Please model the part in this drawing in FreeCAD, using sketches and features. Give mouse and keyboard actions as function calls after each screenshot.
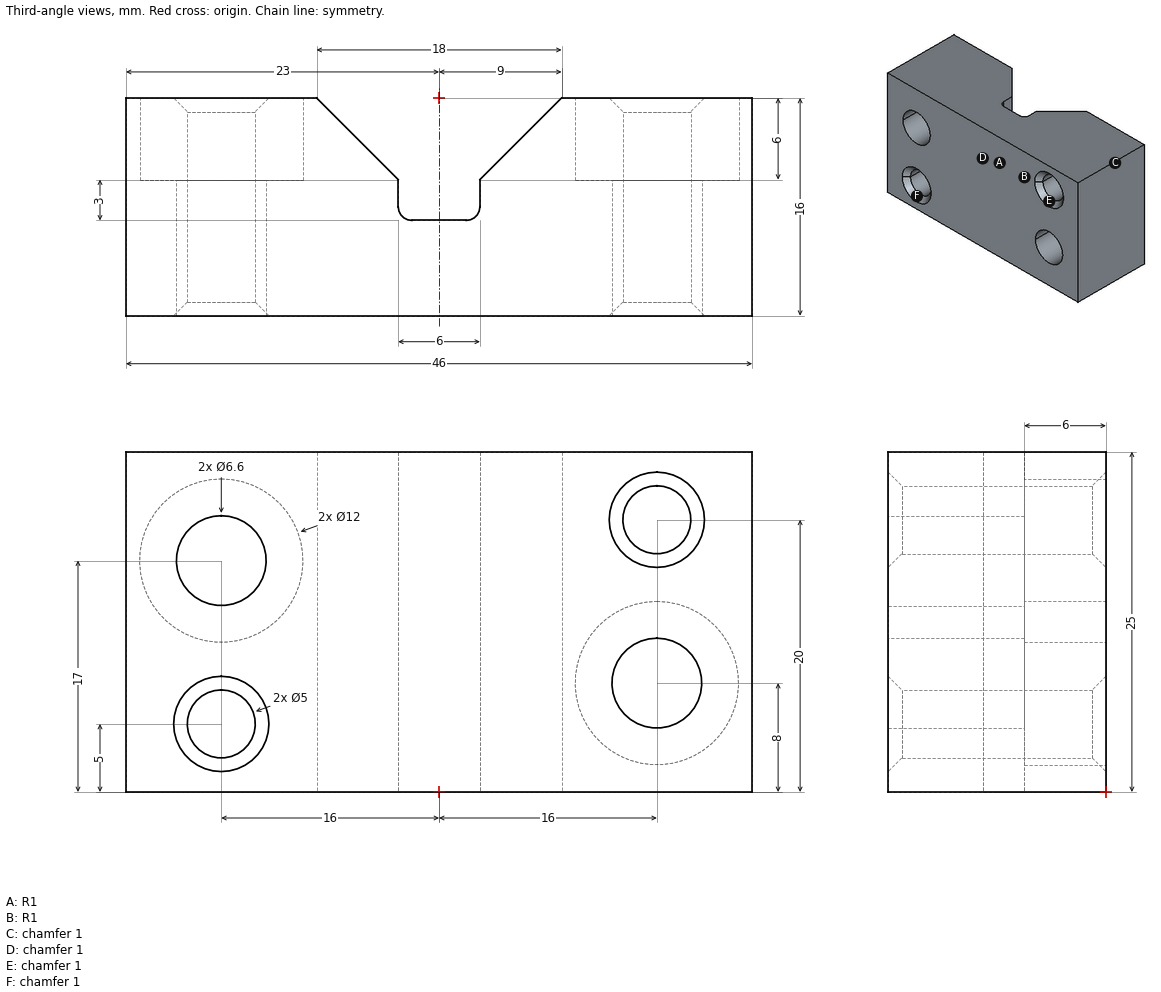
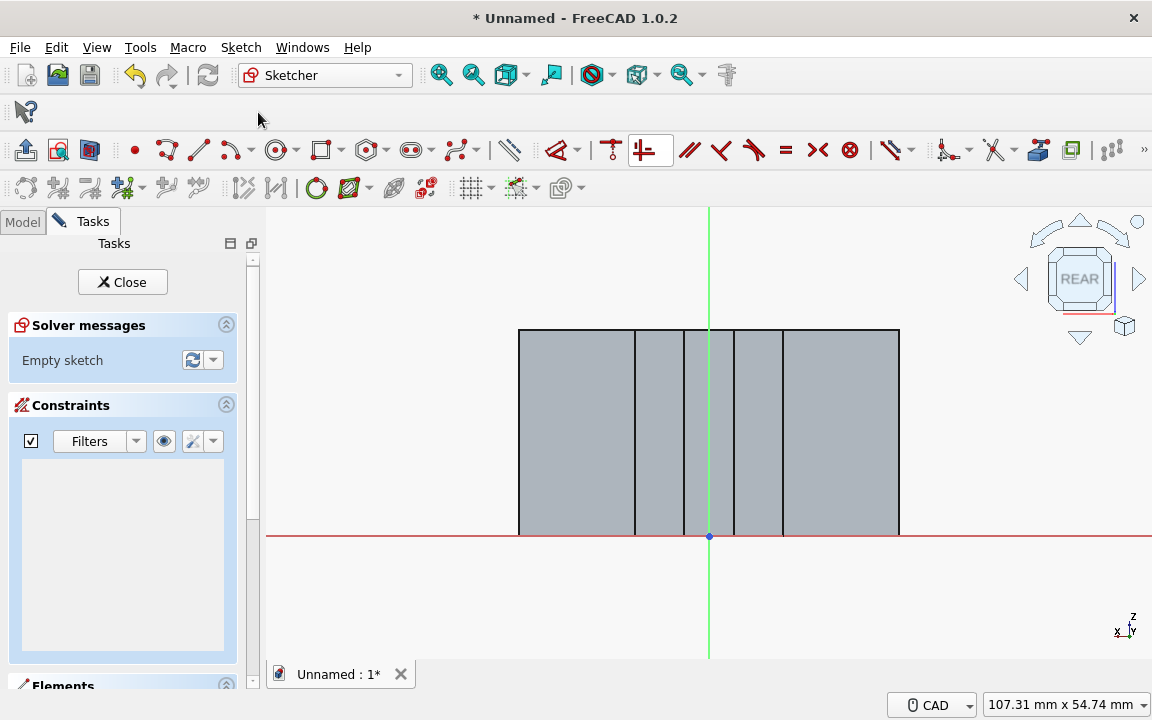
scroll(848, 464, up, 2)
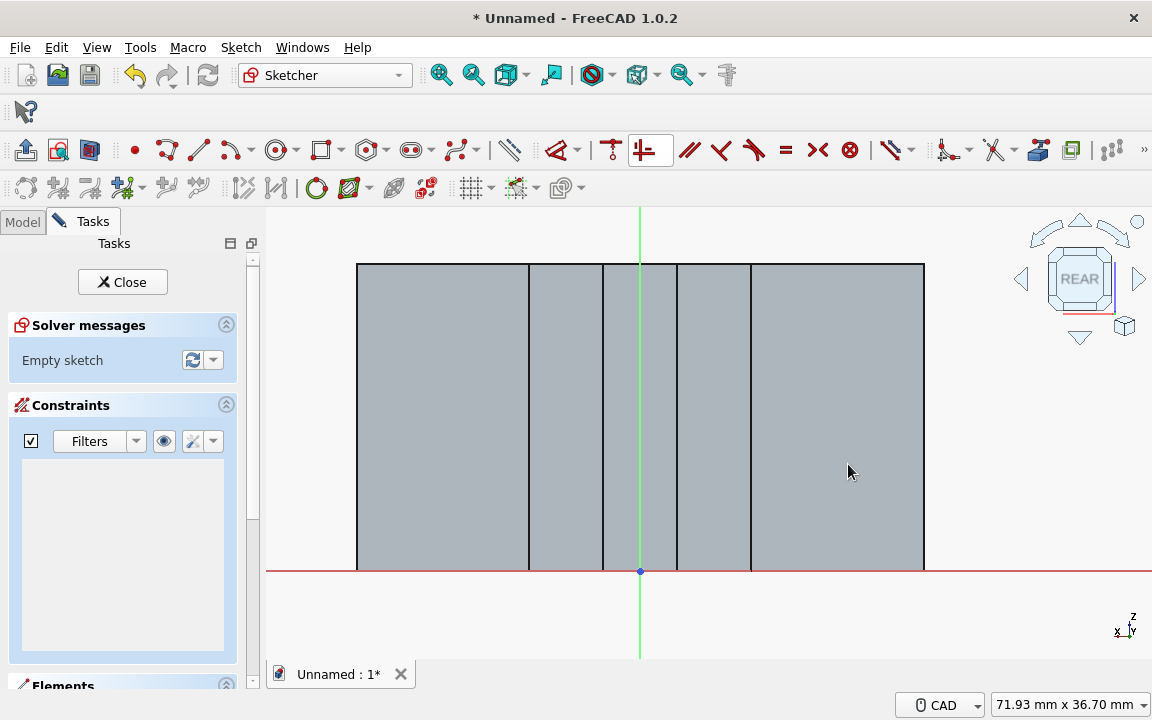
click(276, 150)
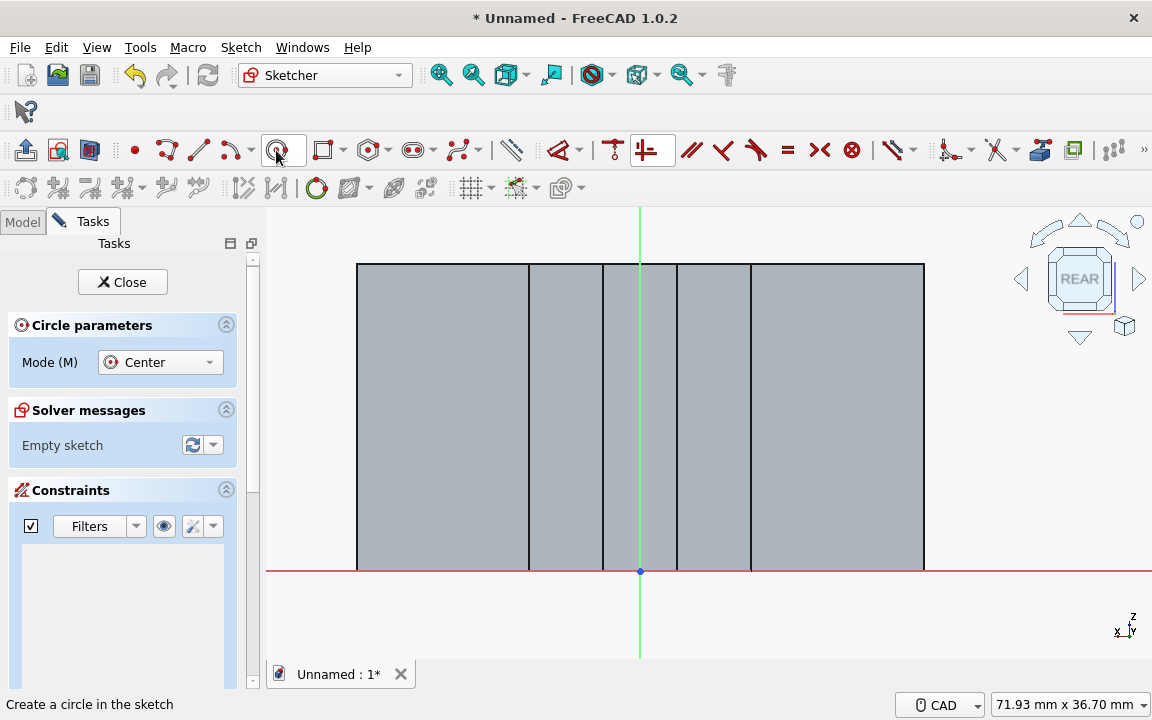
click(837, 362)
move(866, 333)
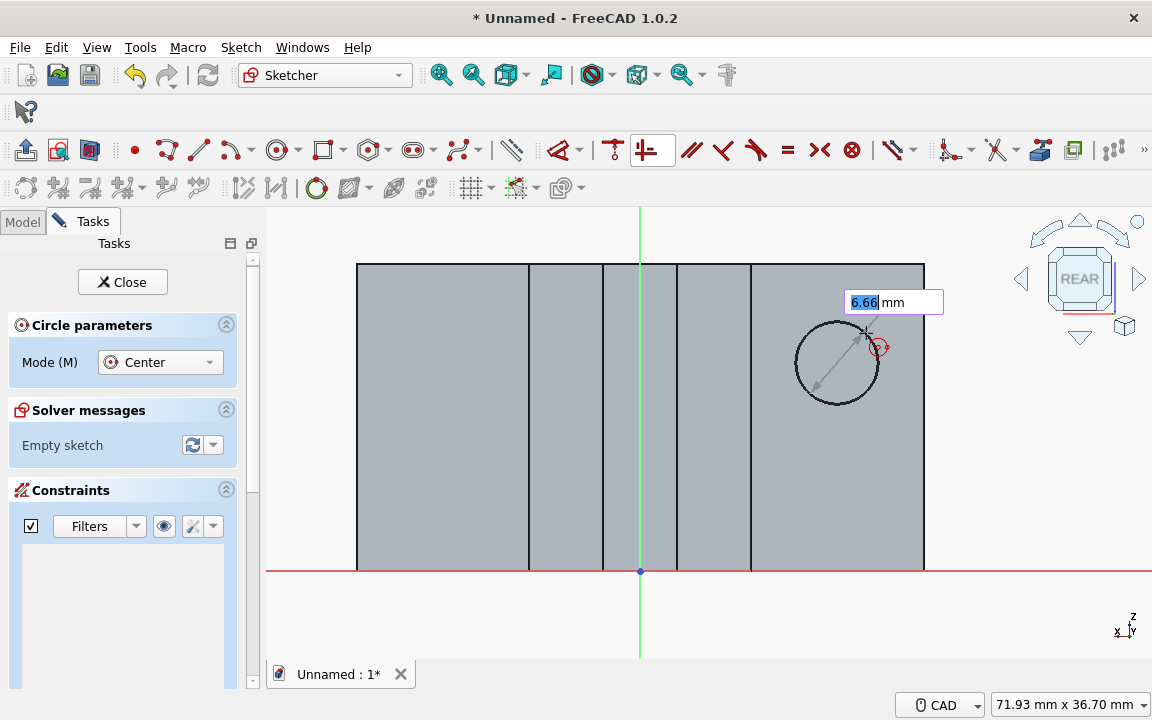
text(6.6)
key(Return)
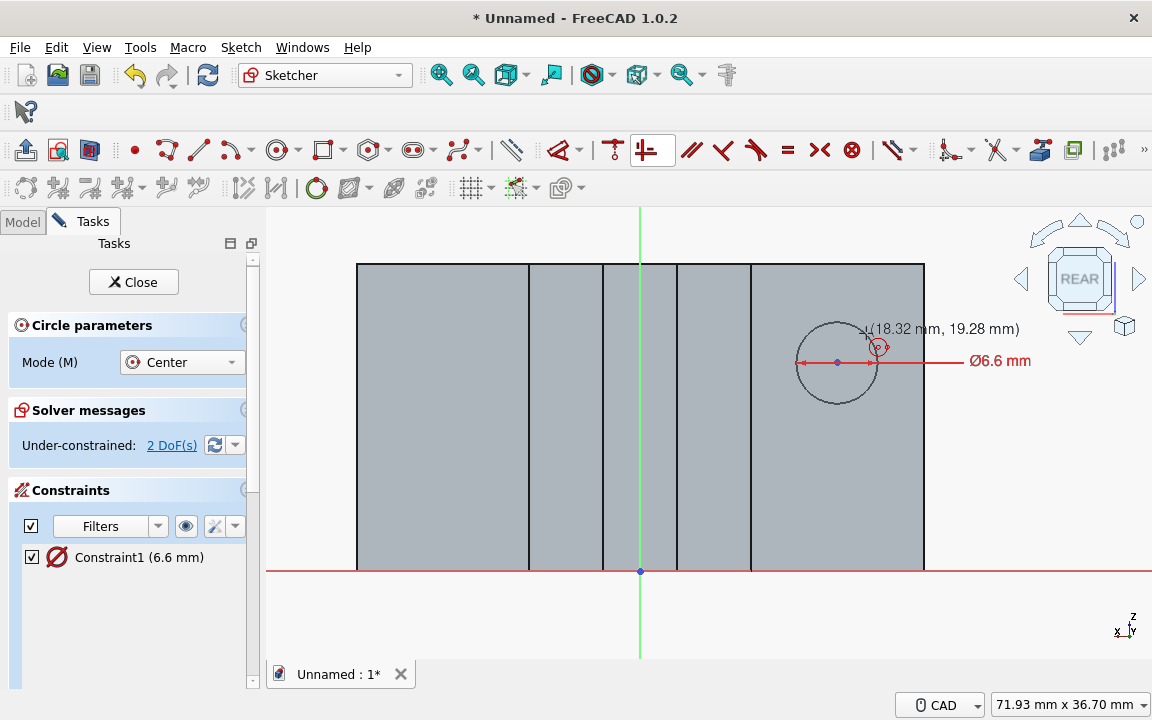
click(837, 510)
move(859, 488)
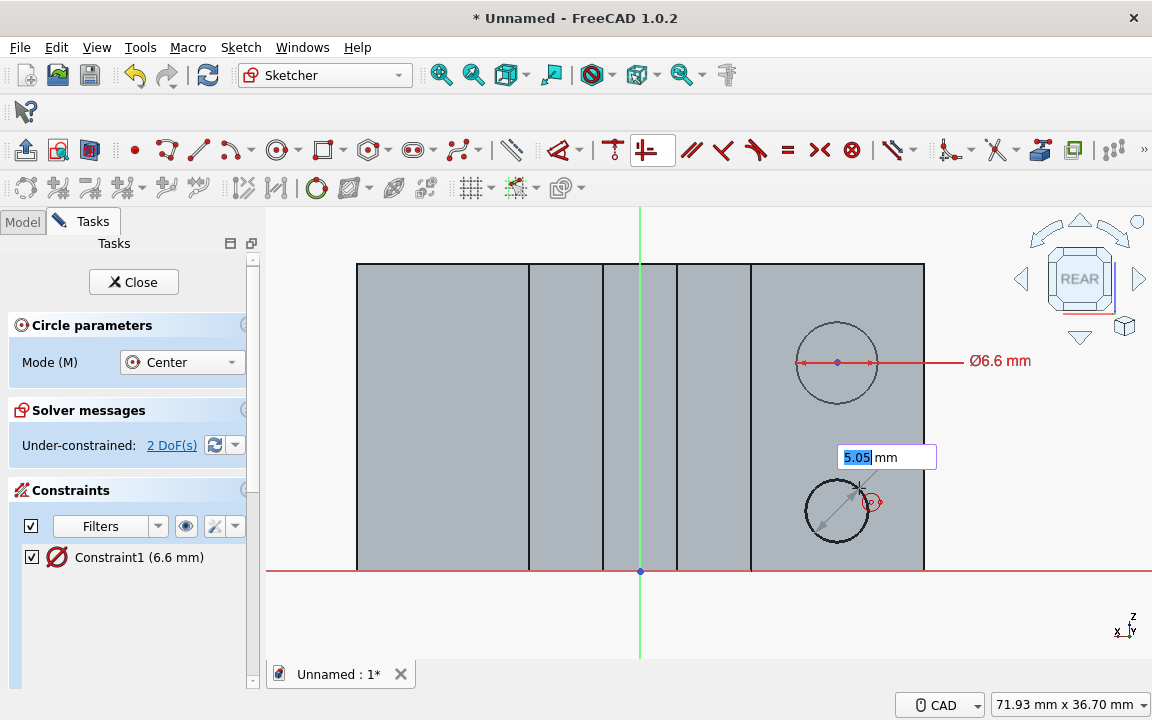
text(5)
key(Return)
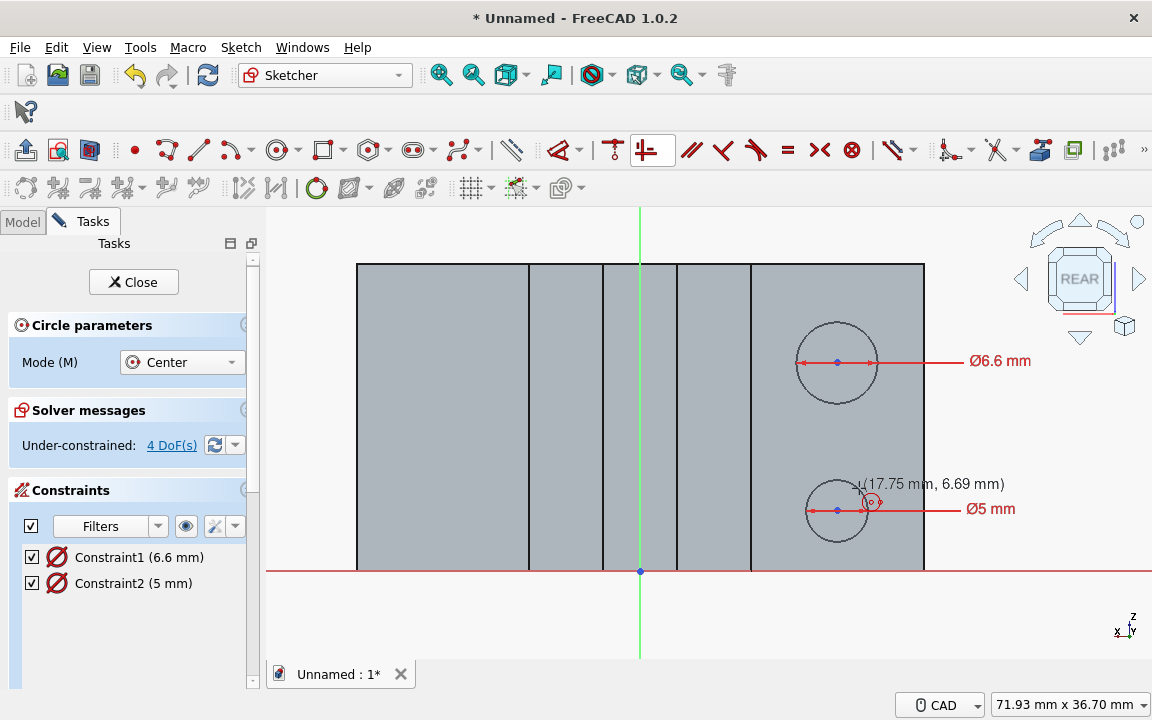
click(443, 325)
move(465, 303)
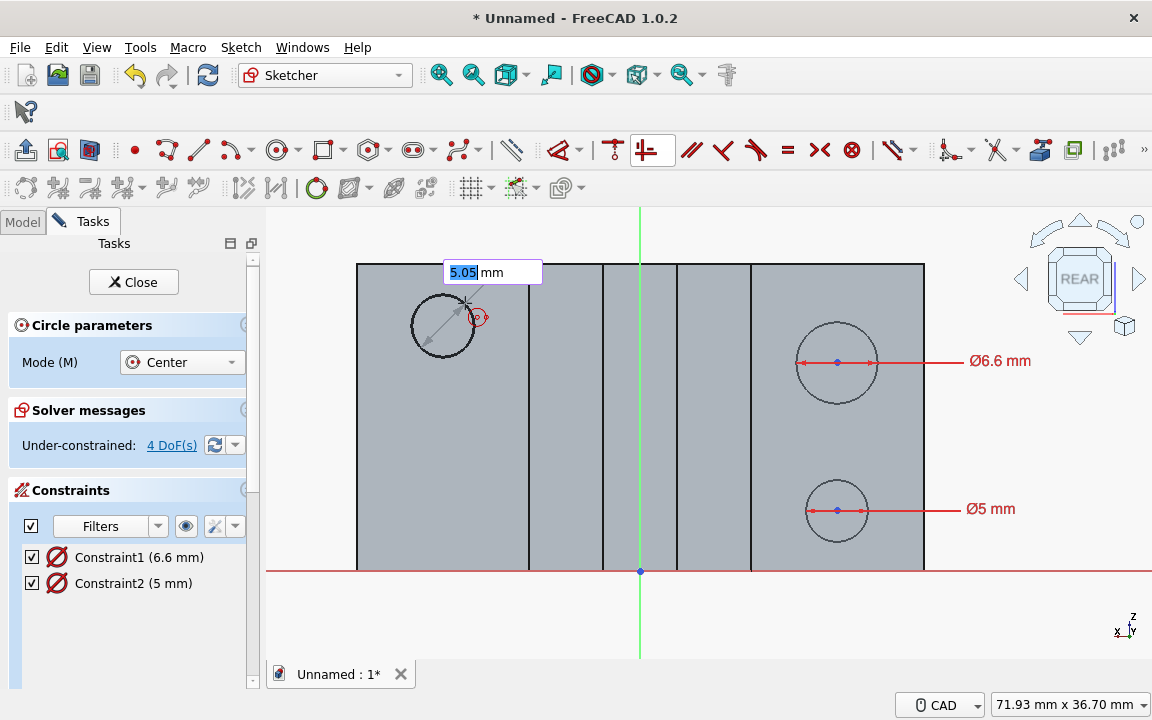
text(5)
key(Return)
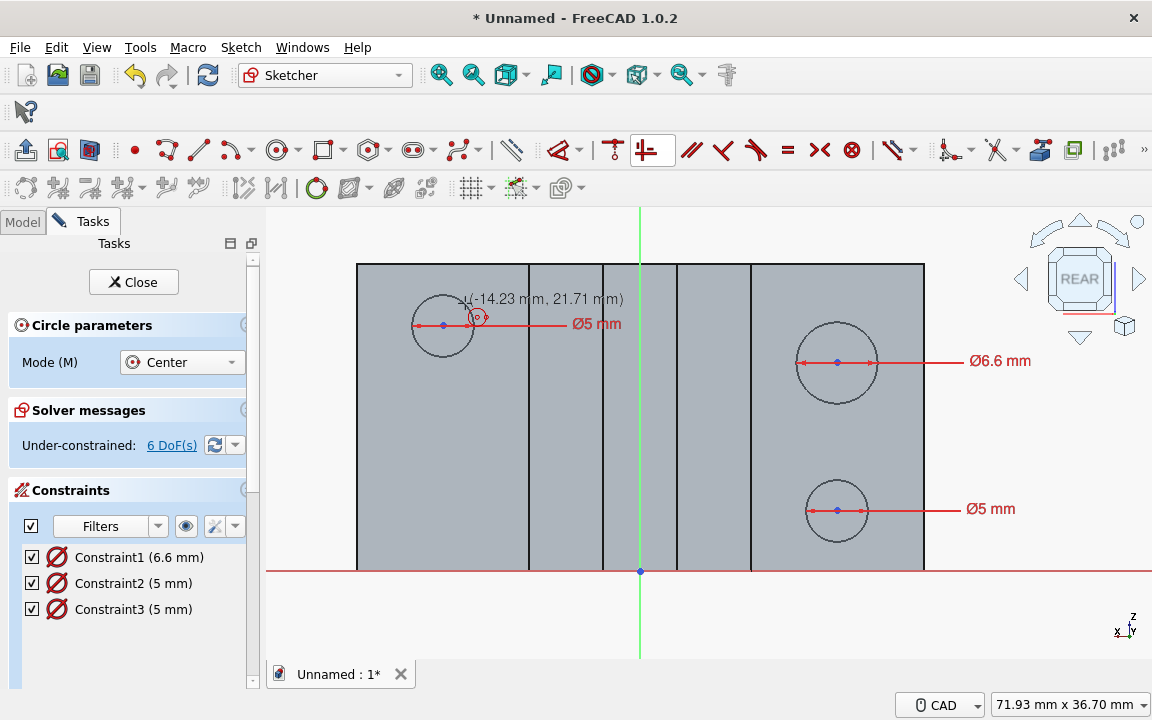
click(443, 473)
move(472, 444)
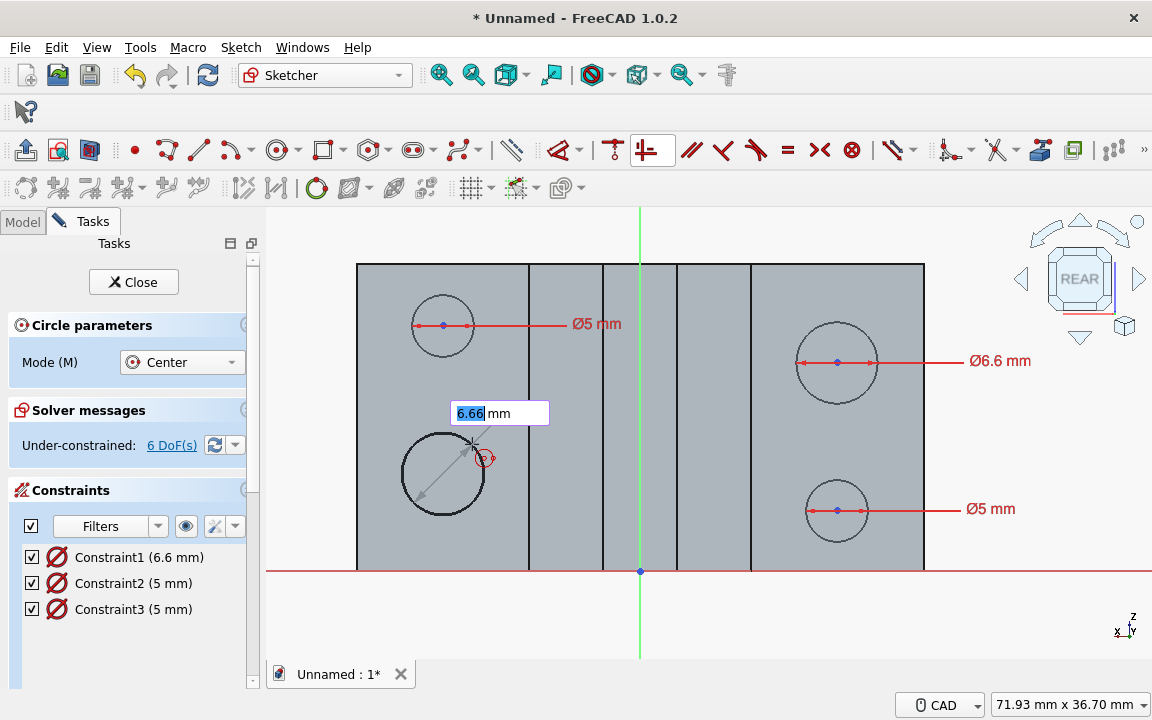
text(6.6)
key(Return)
key(Escape)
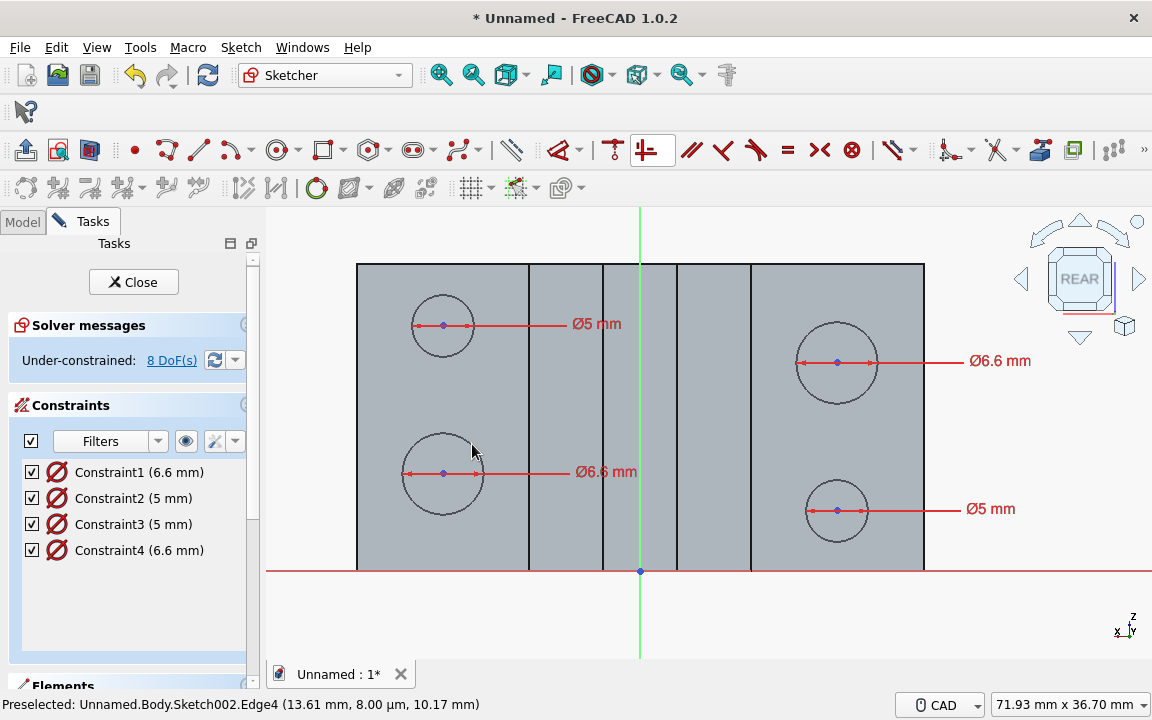
click(837, 511)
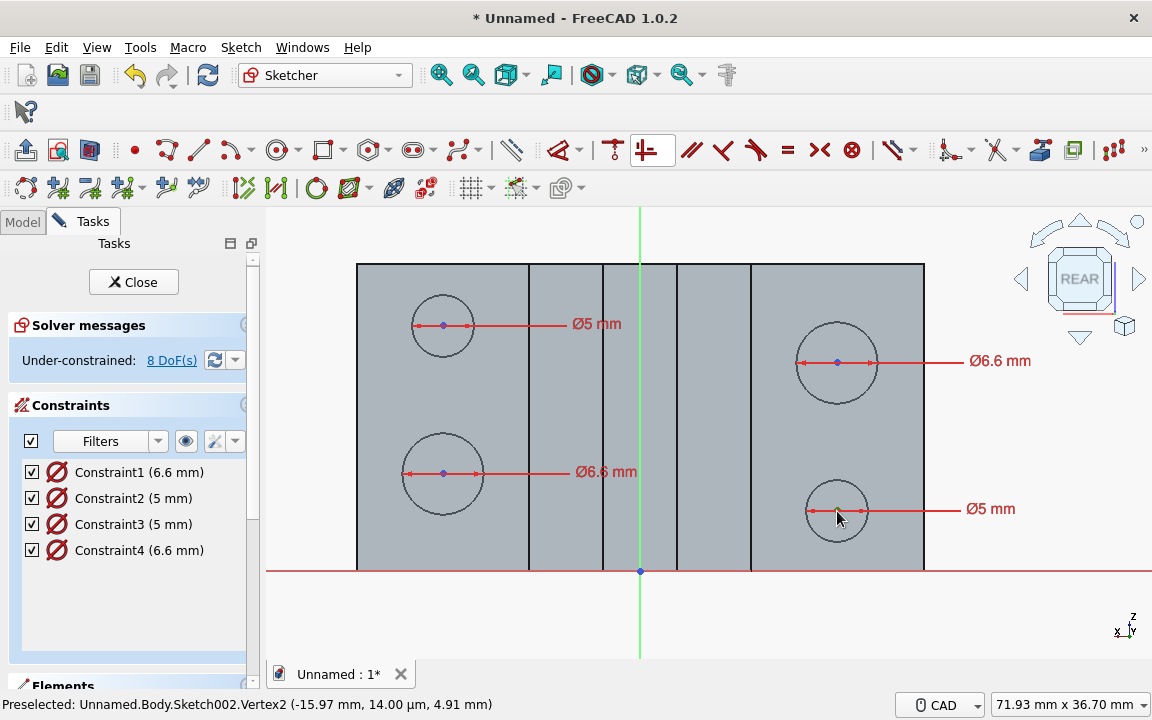
key(i)